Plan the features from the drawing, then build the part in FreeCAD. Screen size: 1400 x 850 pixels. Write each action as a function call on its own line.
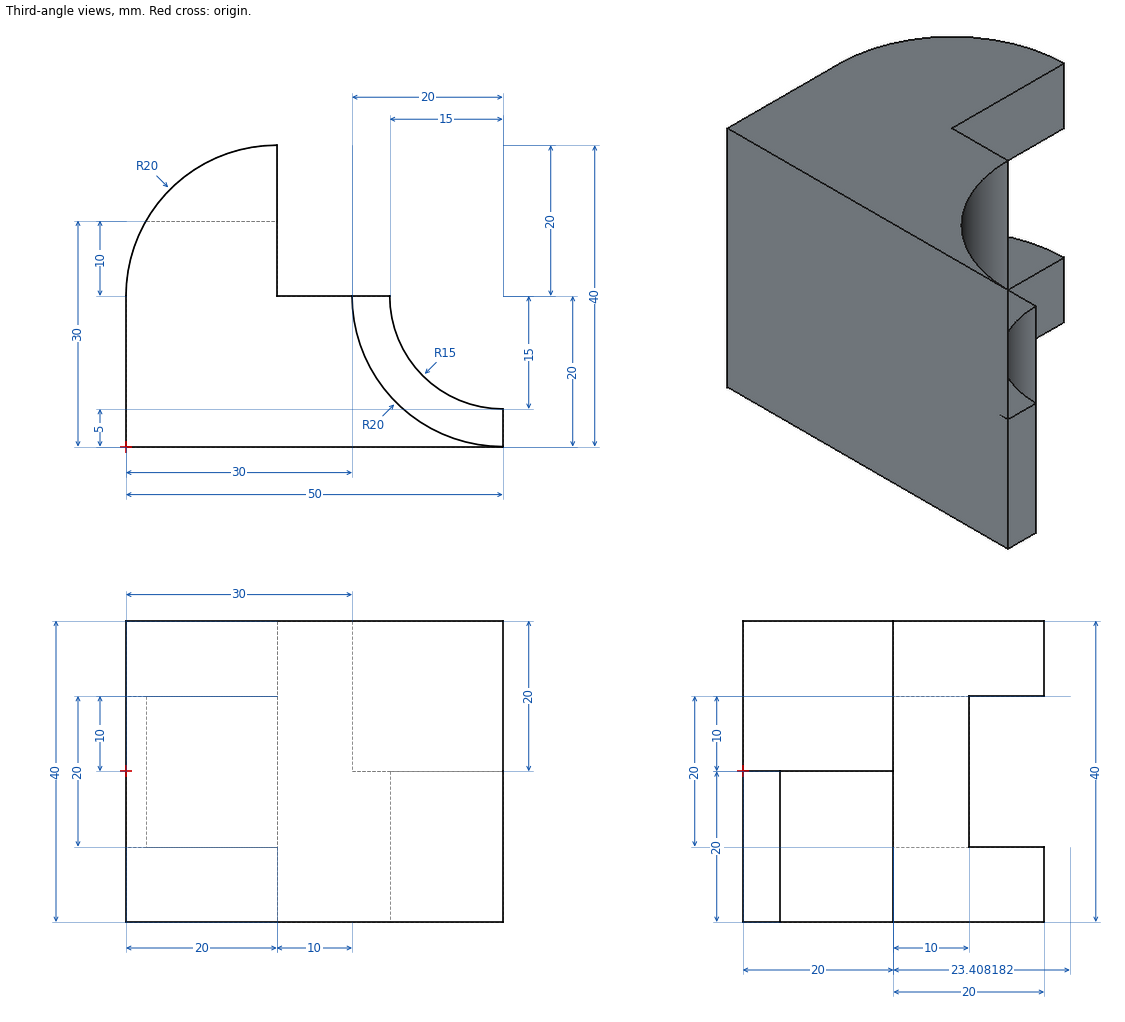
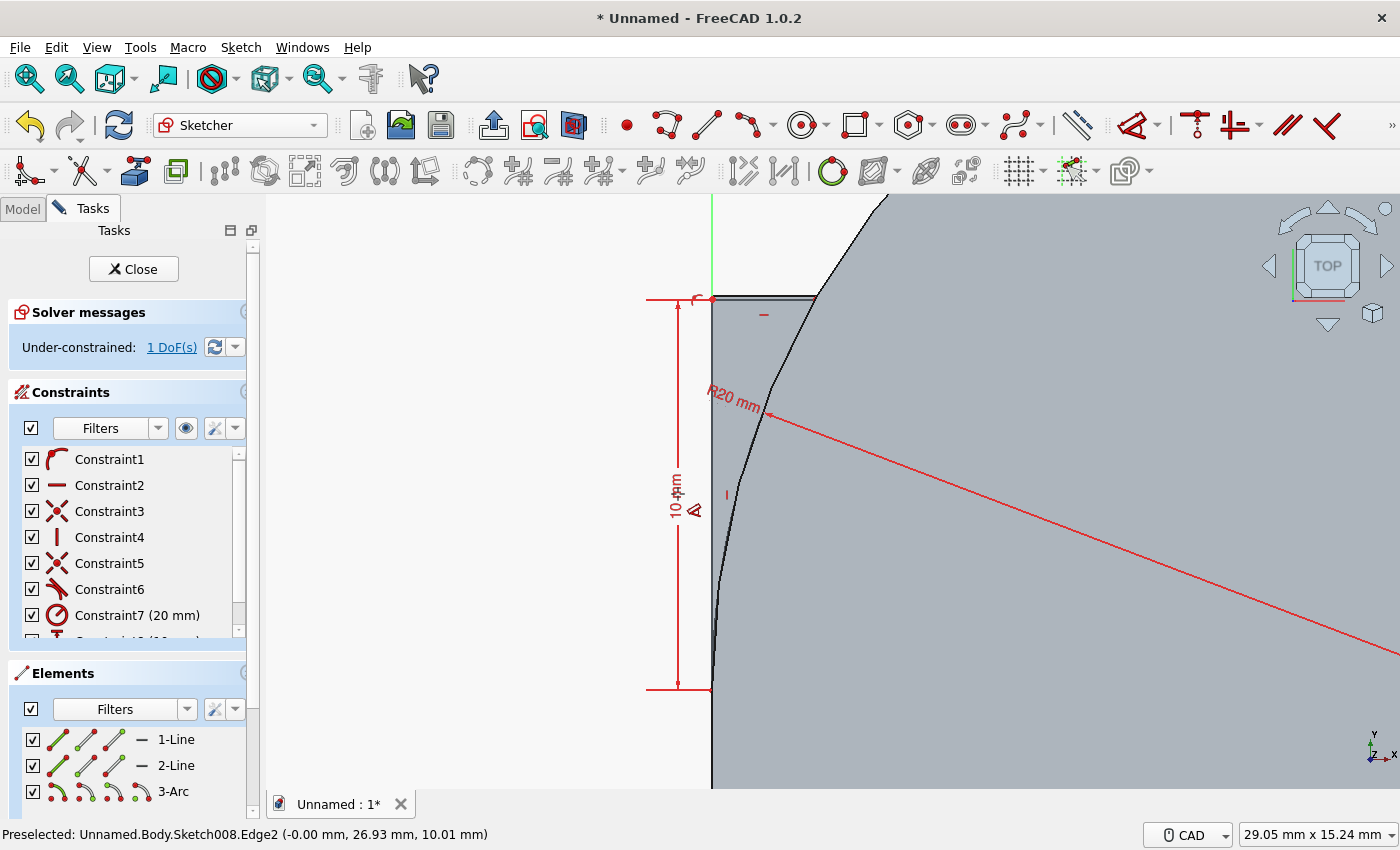
click(817, 300)
click(851, 530)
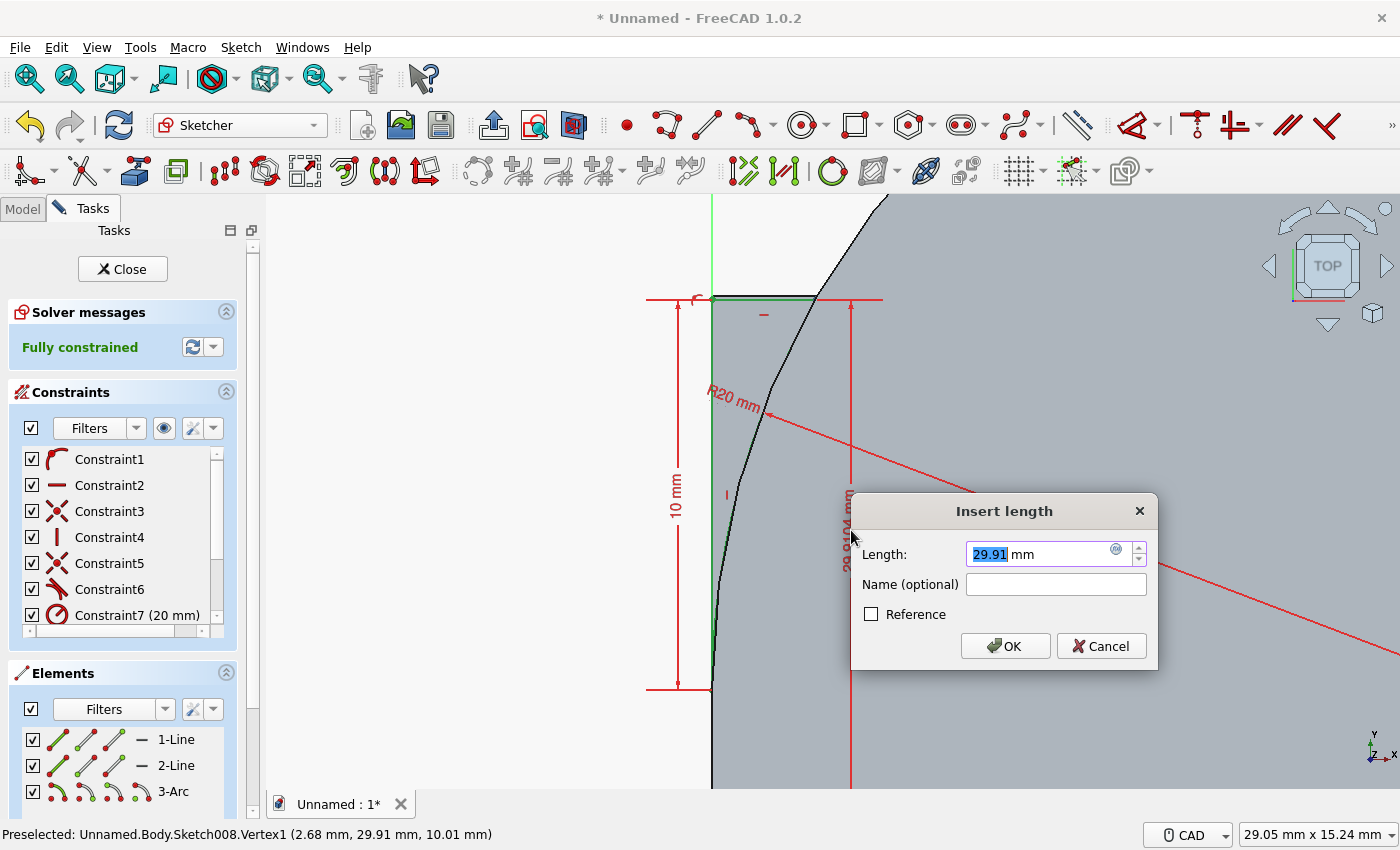
text(30)
key(Return)
key(Escape)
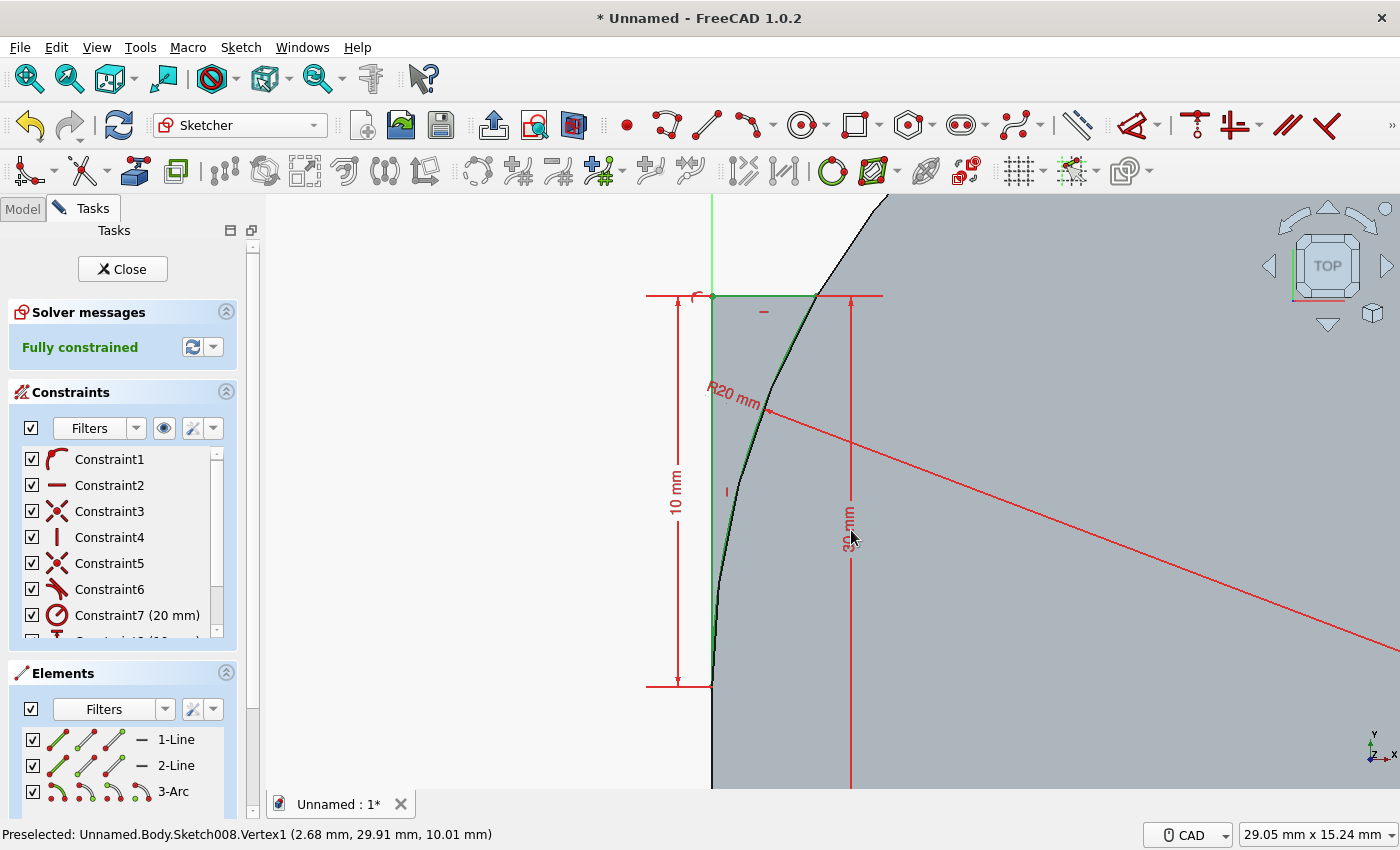
click(123, 269)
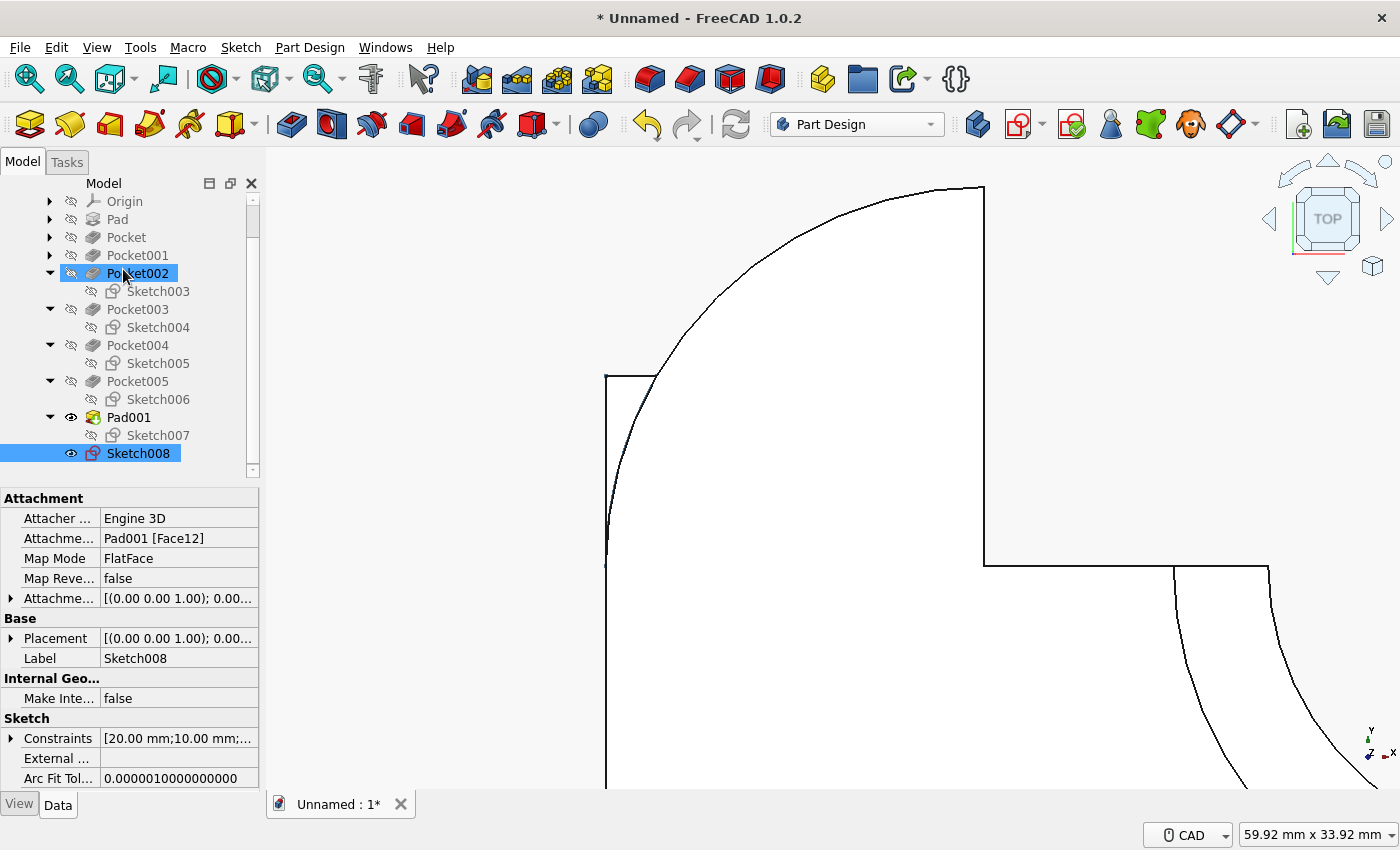
click(292, 124)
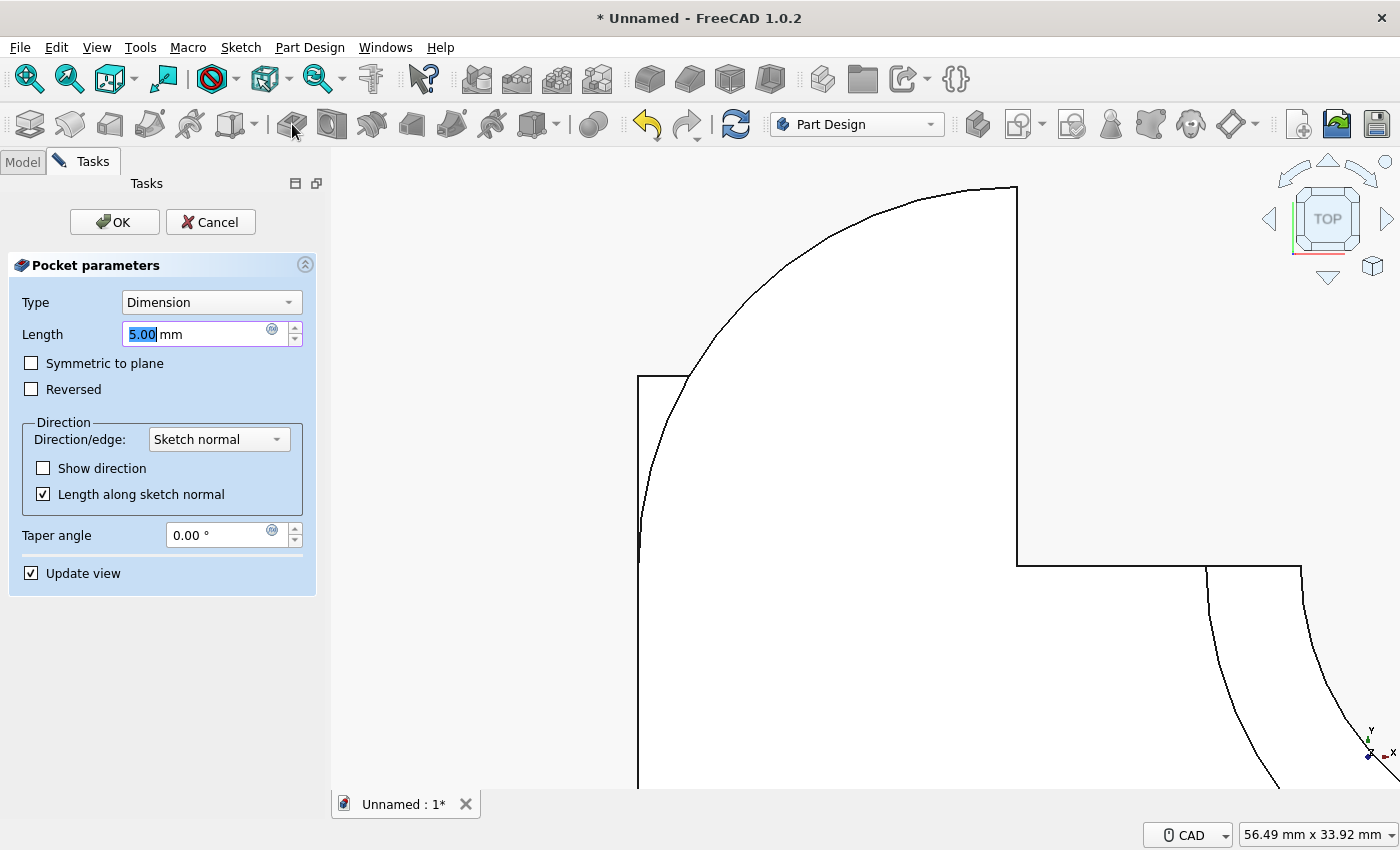
text(20)
key(Tab)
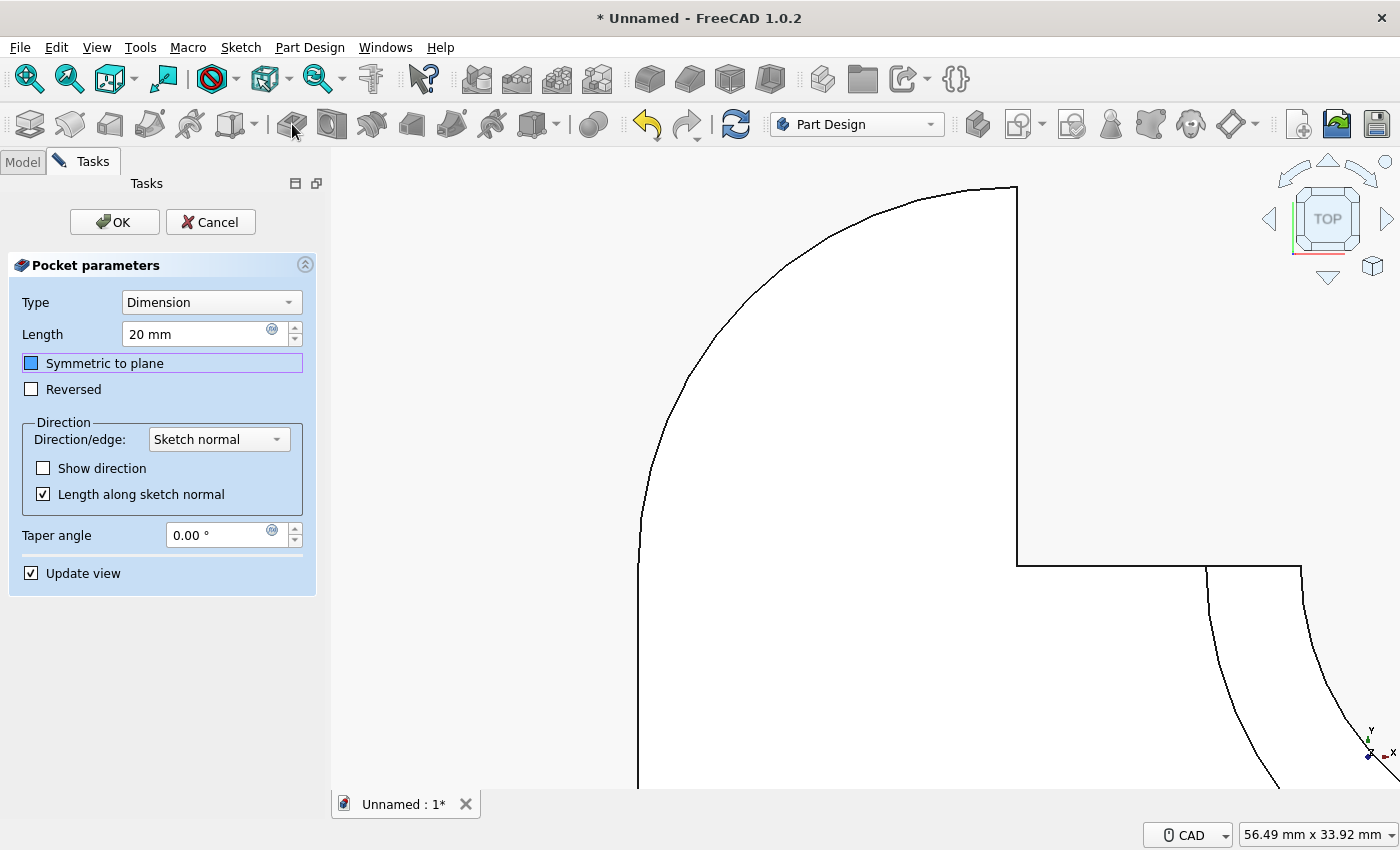
click(115, 222)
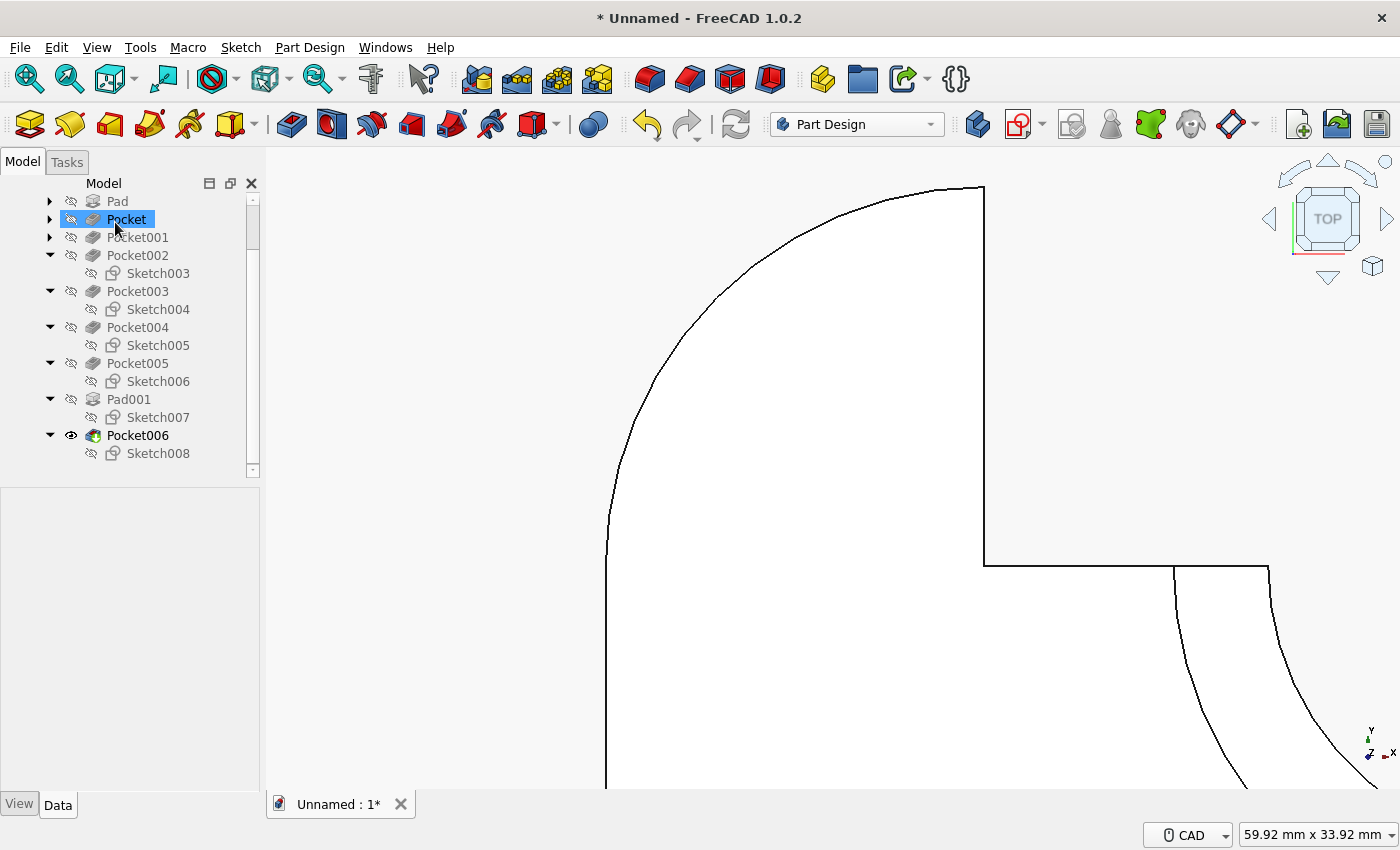
key(0)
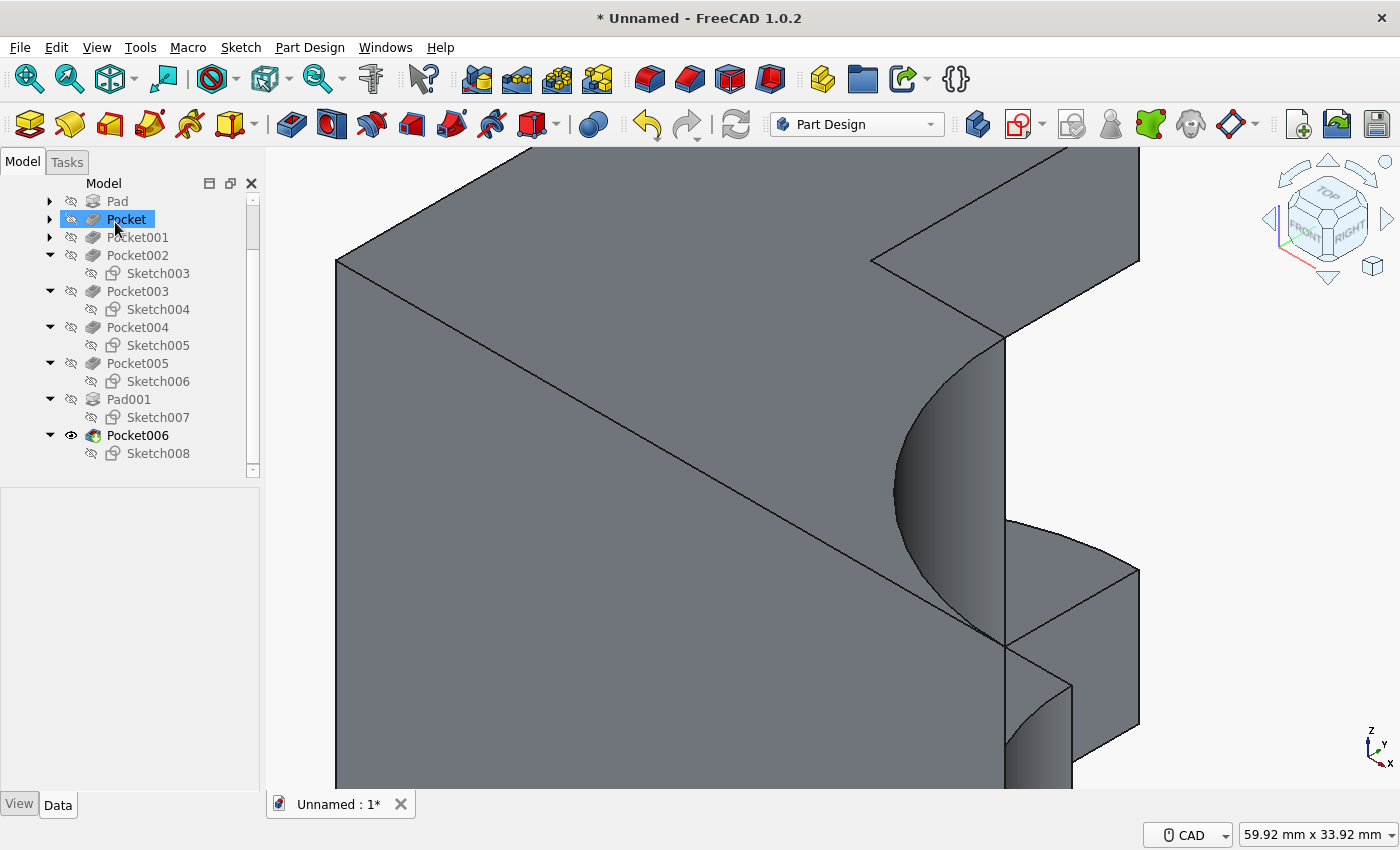
click(30, 80)